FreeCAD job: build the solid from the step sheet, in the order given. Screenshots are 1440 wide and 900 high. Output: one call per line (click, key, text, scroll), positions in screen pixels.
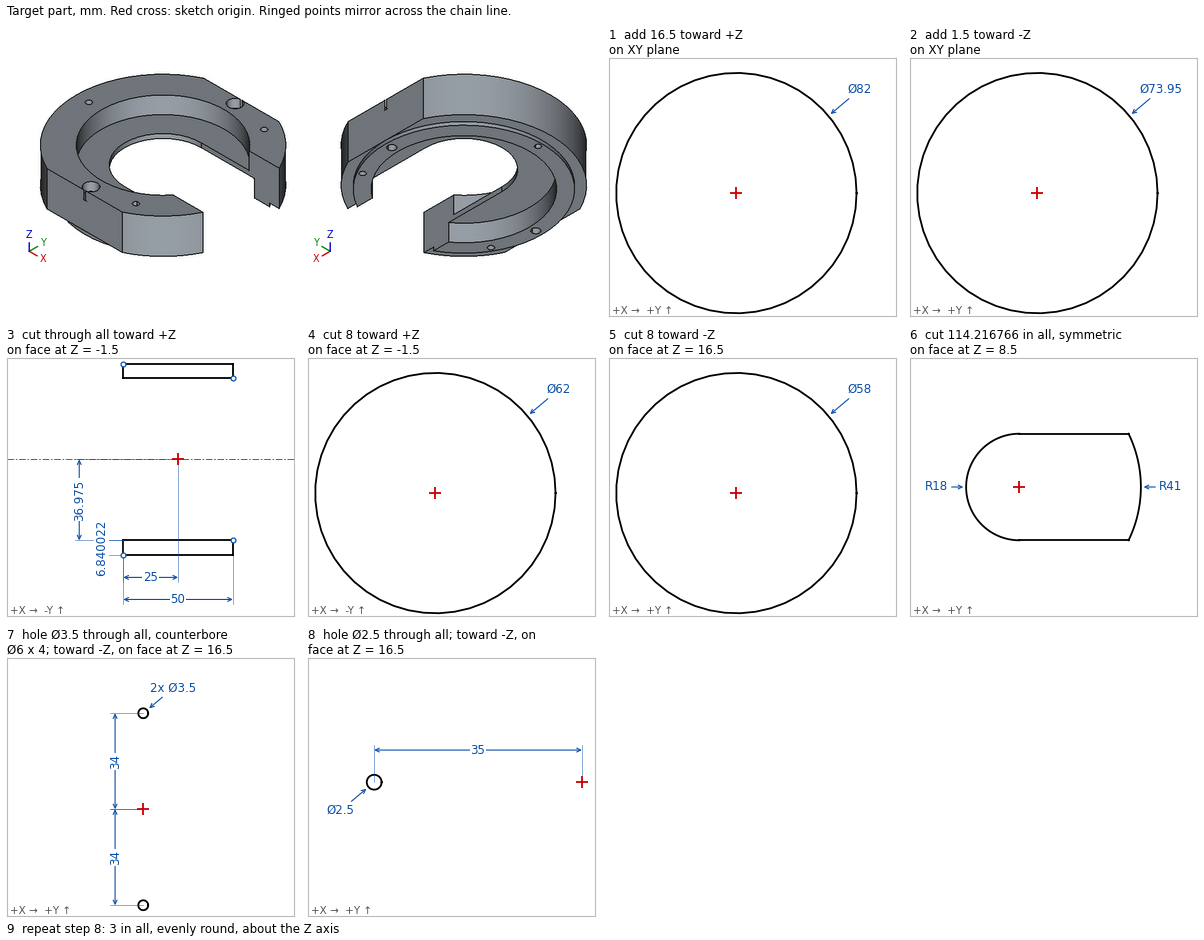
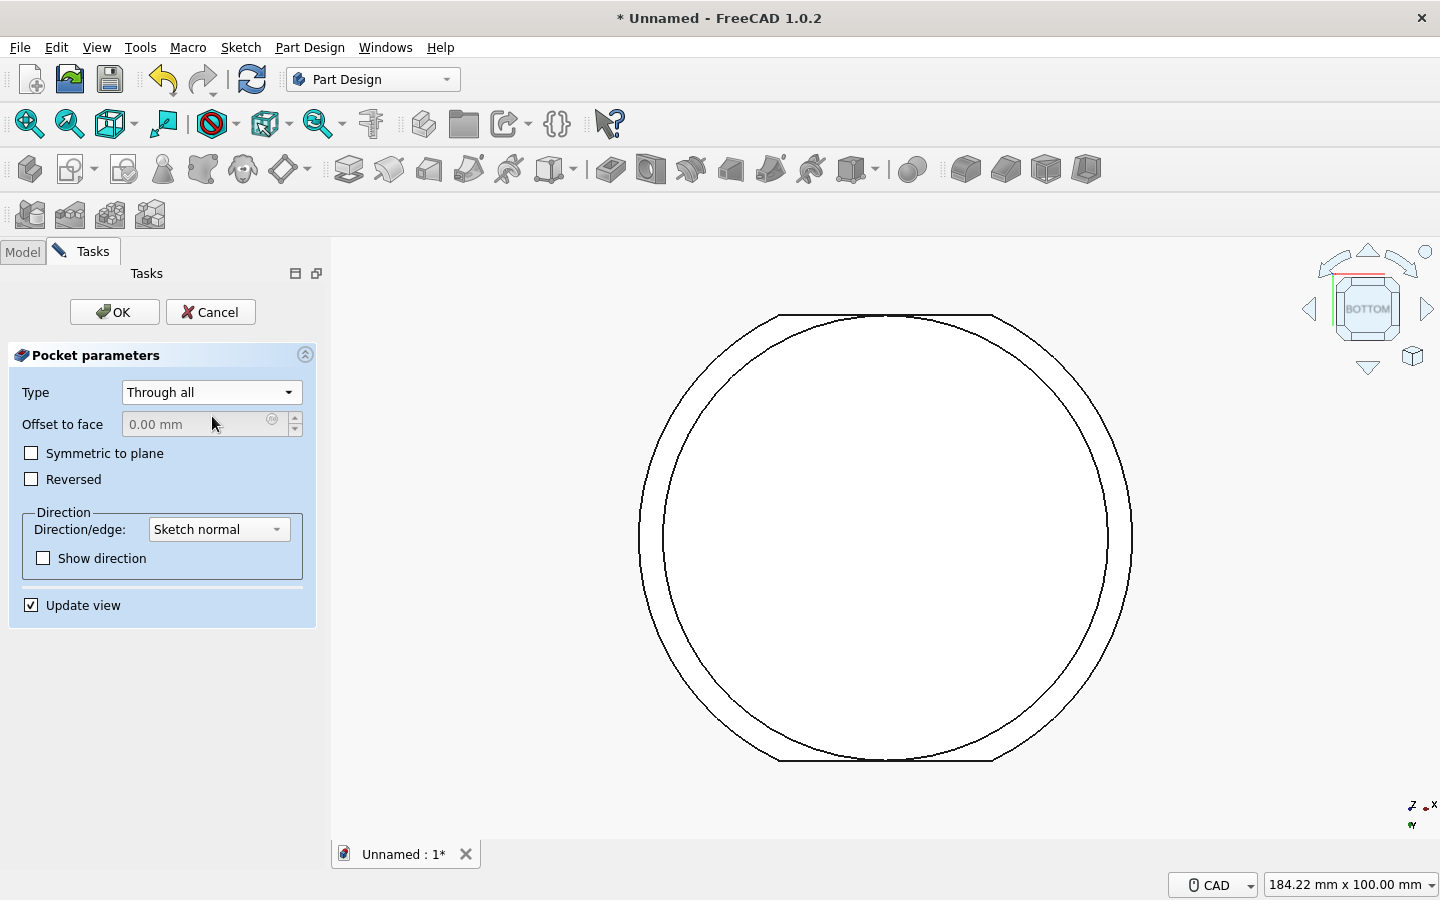
click(115, 312)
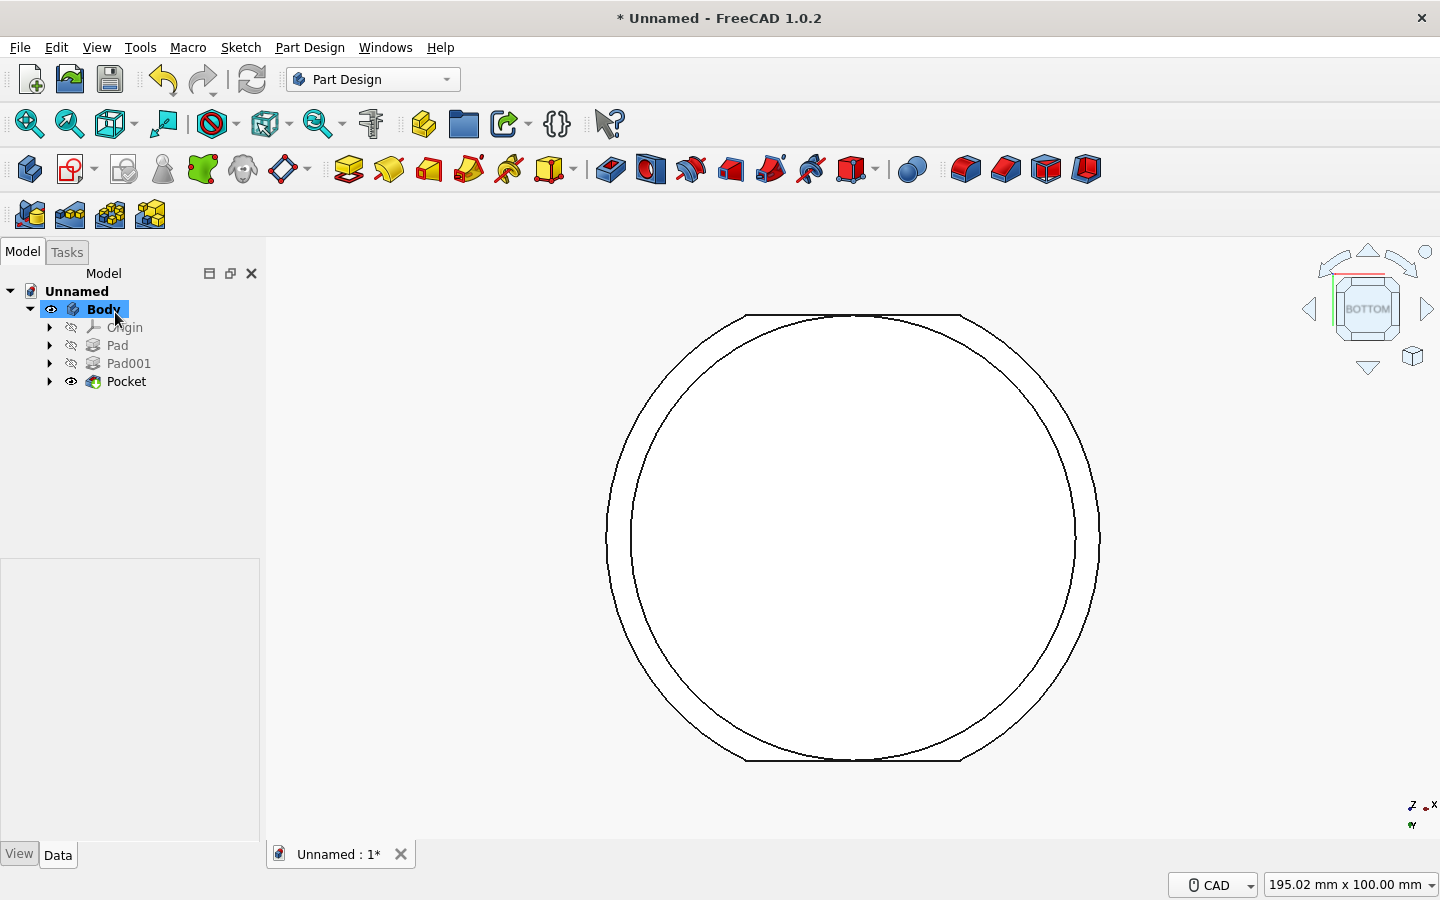
click(853, 537)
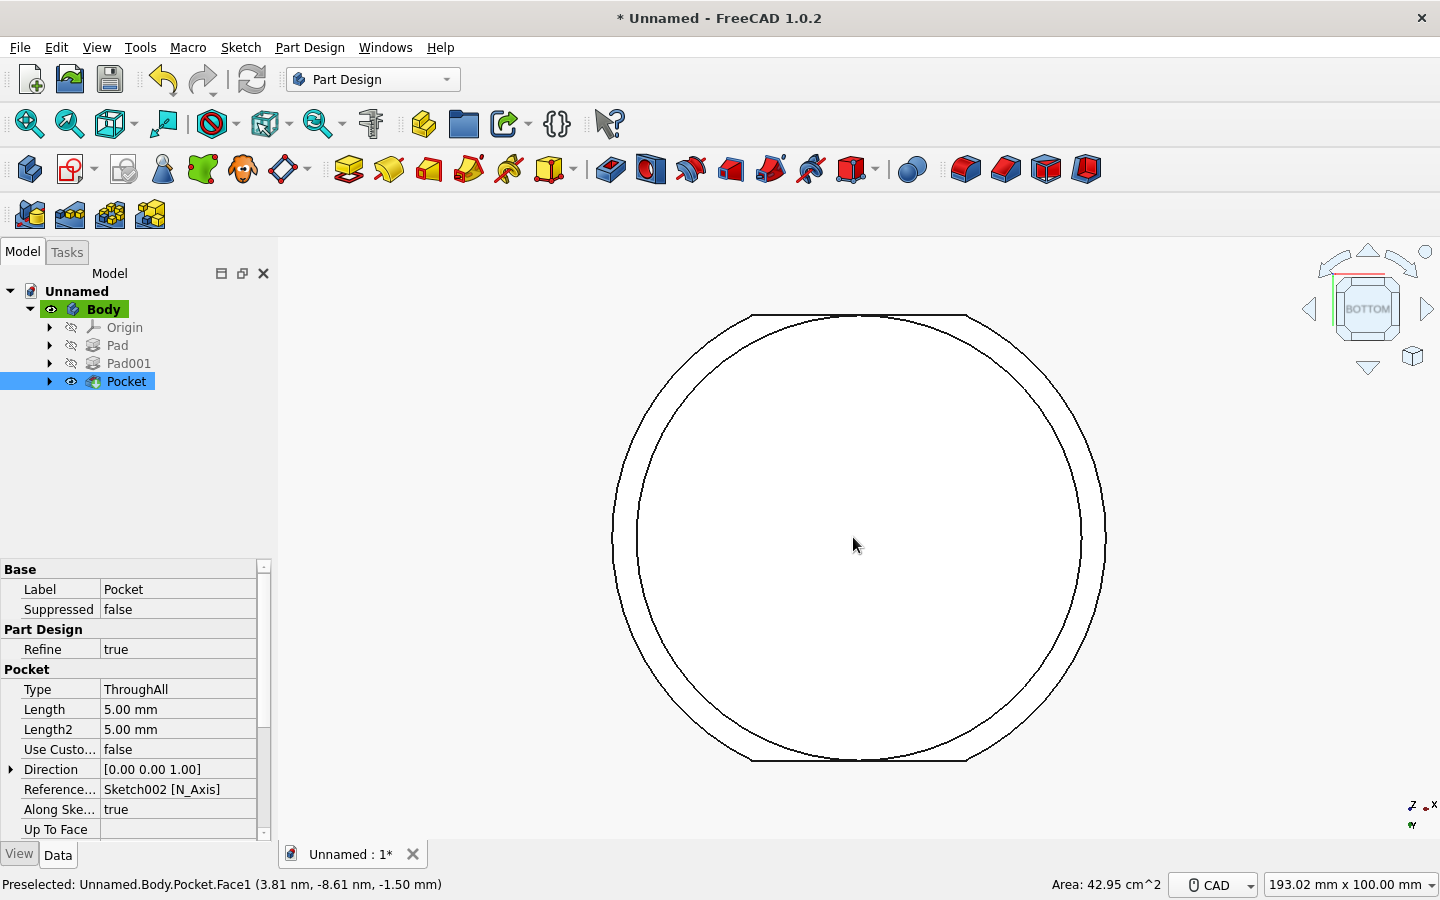
click(70, 170)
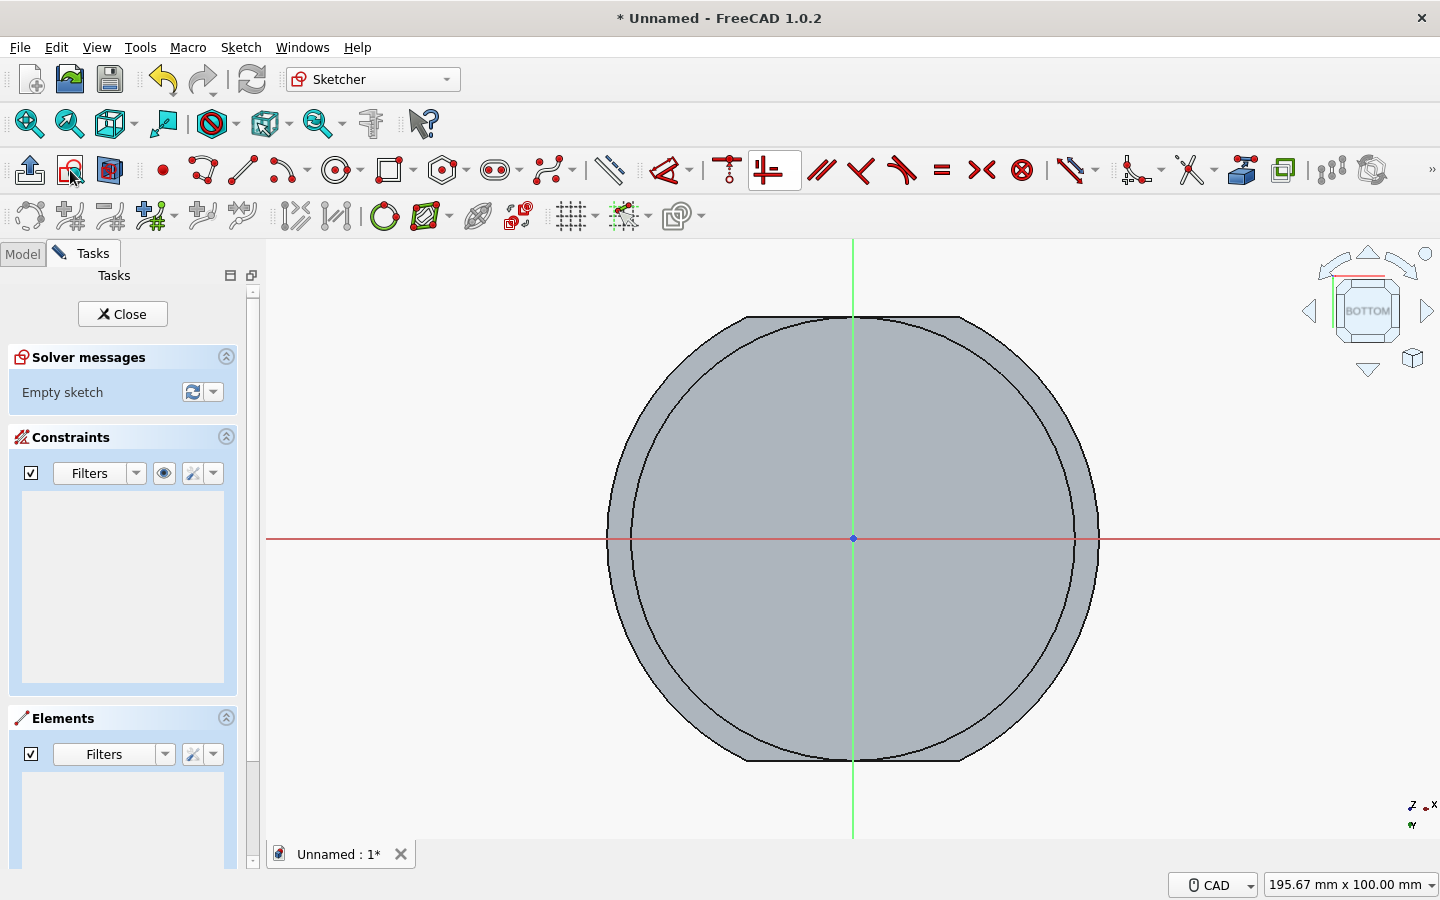
key(g)
key(c)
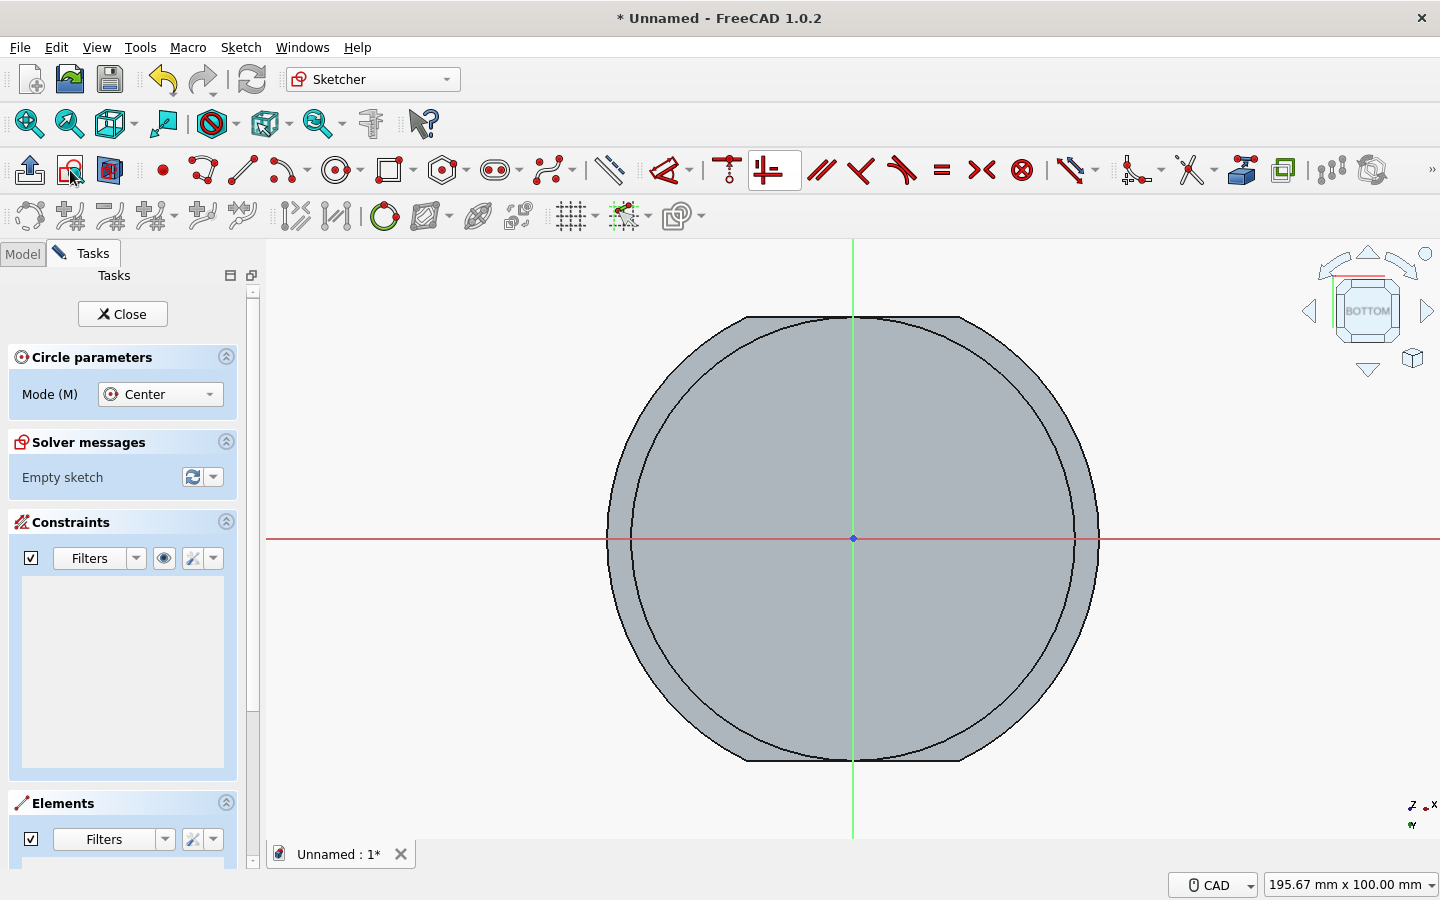
click(853, 539)
click(985, 407)
key(Escape)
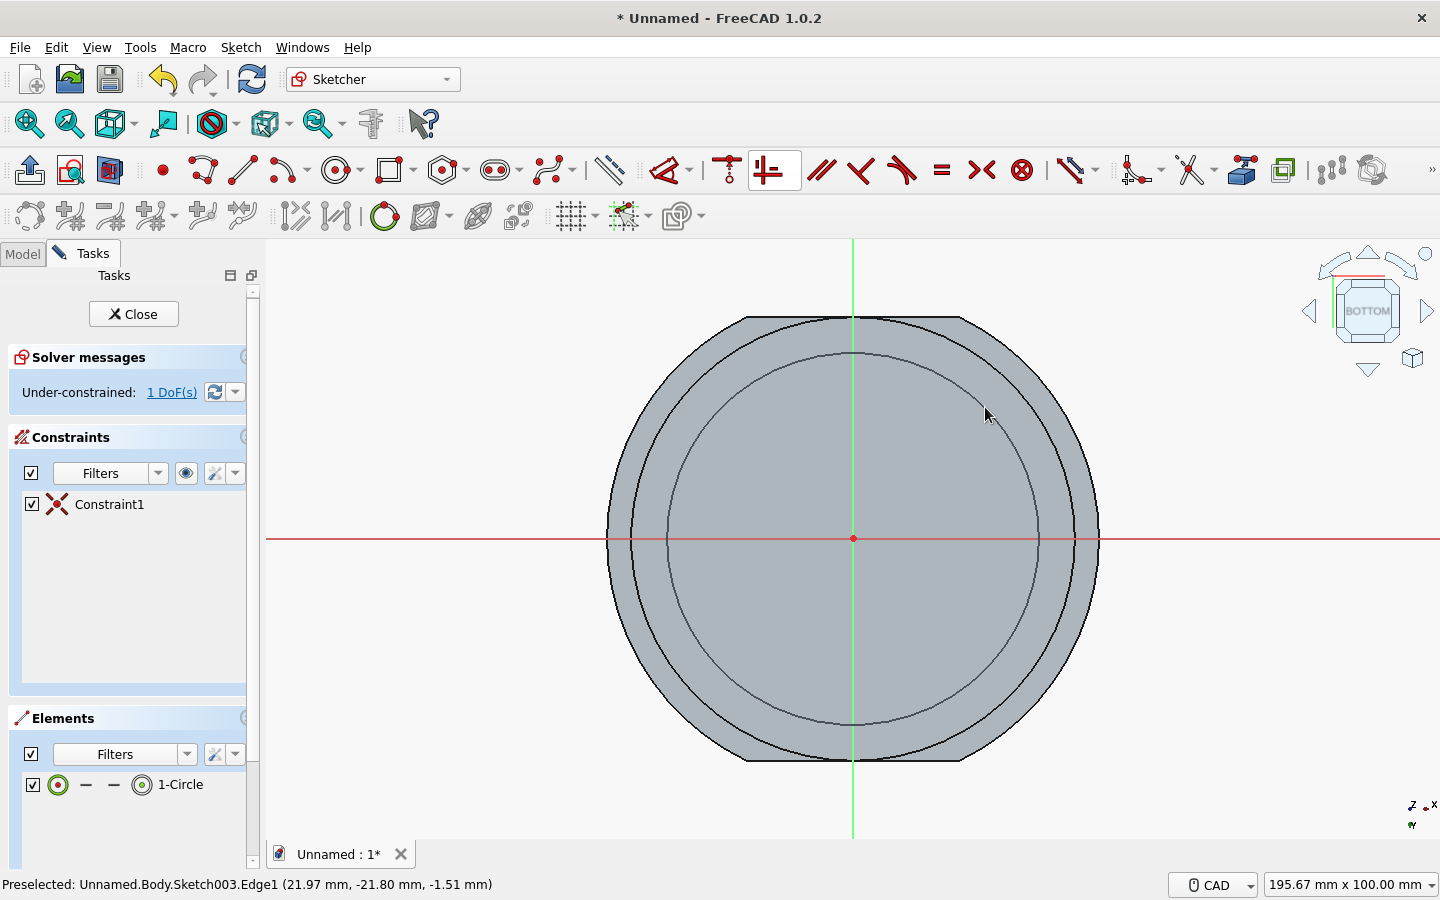
key(d)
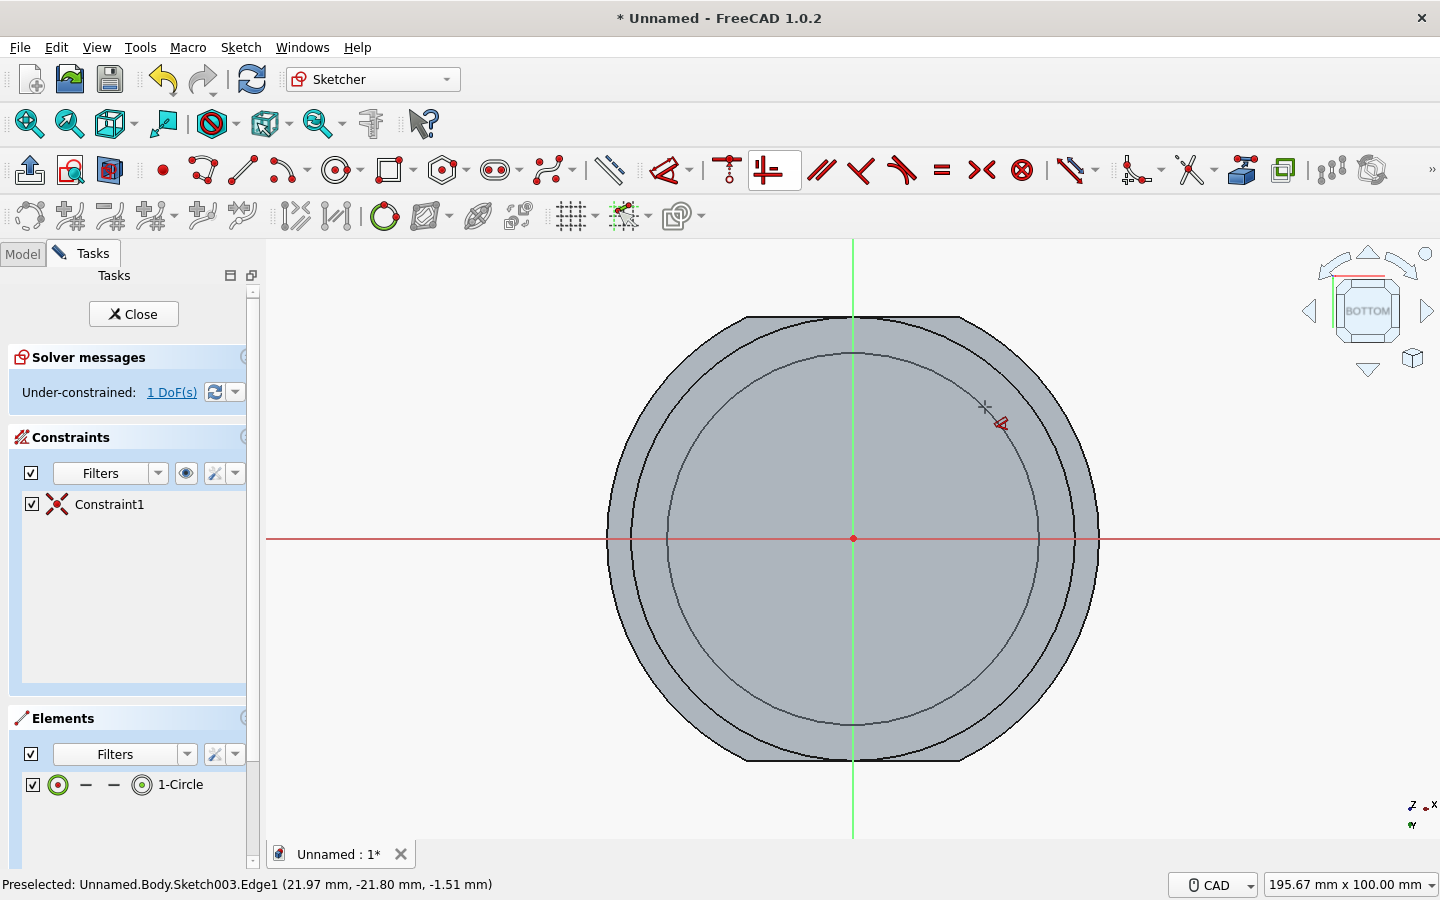
click(984, 407)
click(1007, 384)